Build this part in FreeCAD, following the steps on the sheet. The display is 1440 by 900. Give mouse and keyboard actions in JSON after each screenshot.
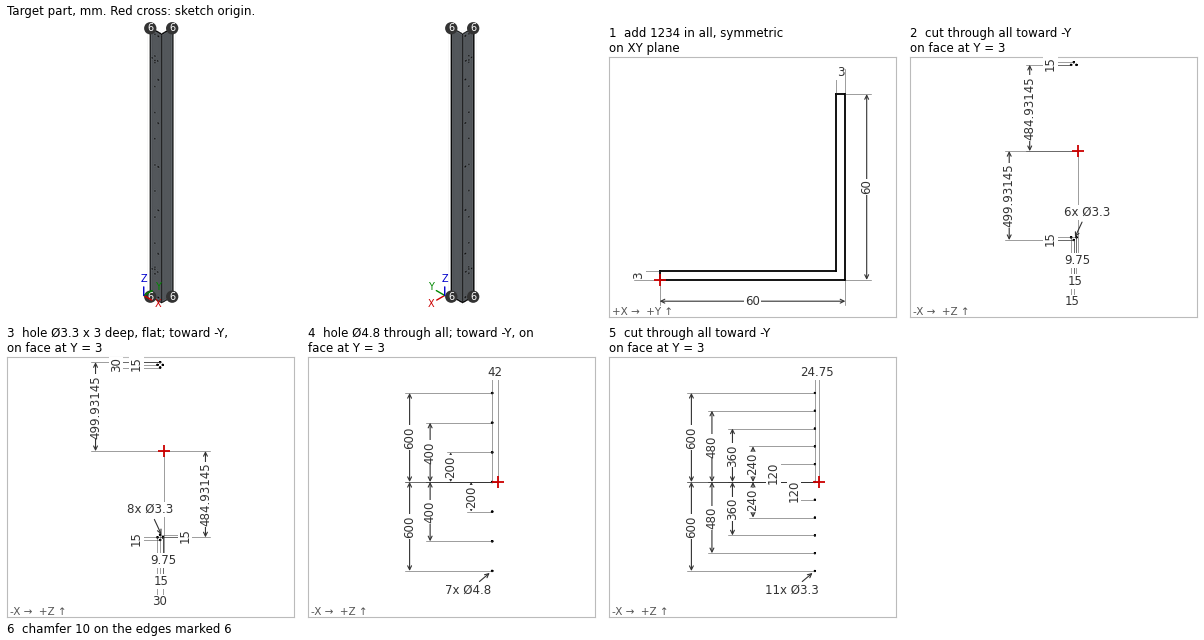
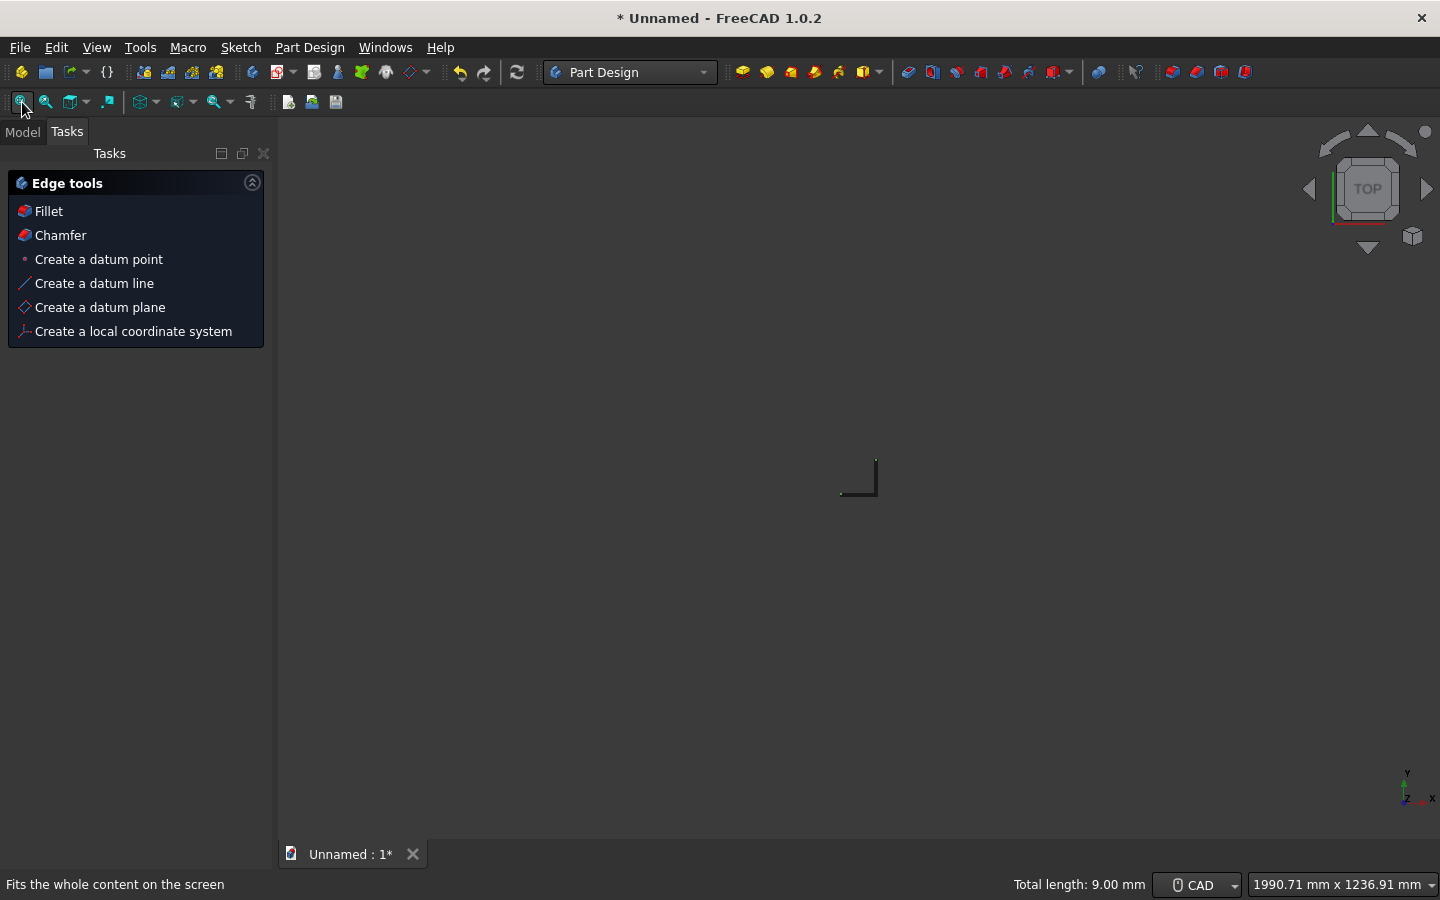
{"action": "left_click", "coordinate": [22, 102]}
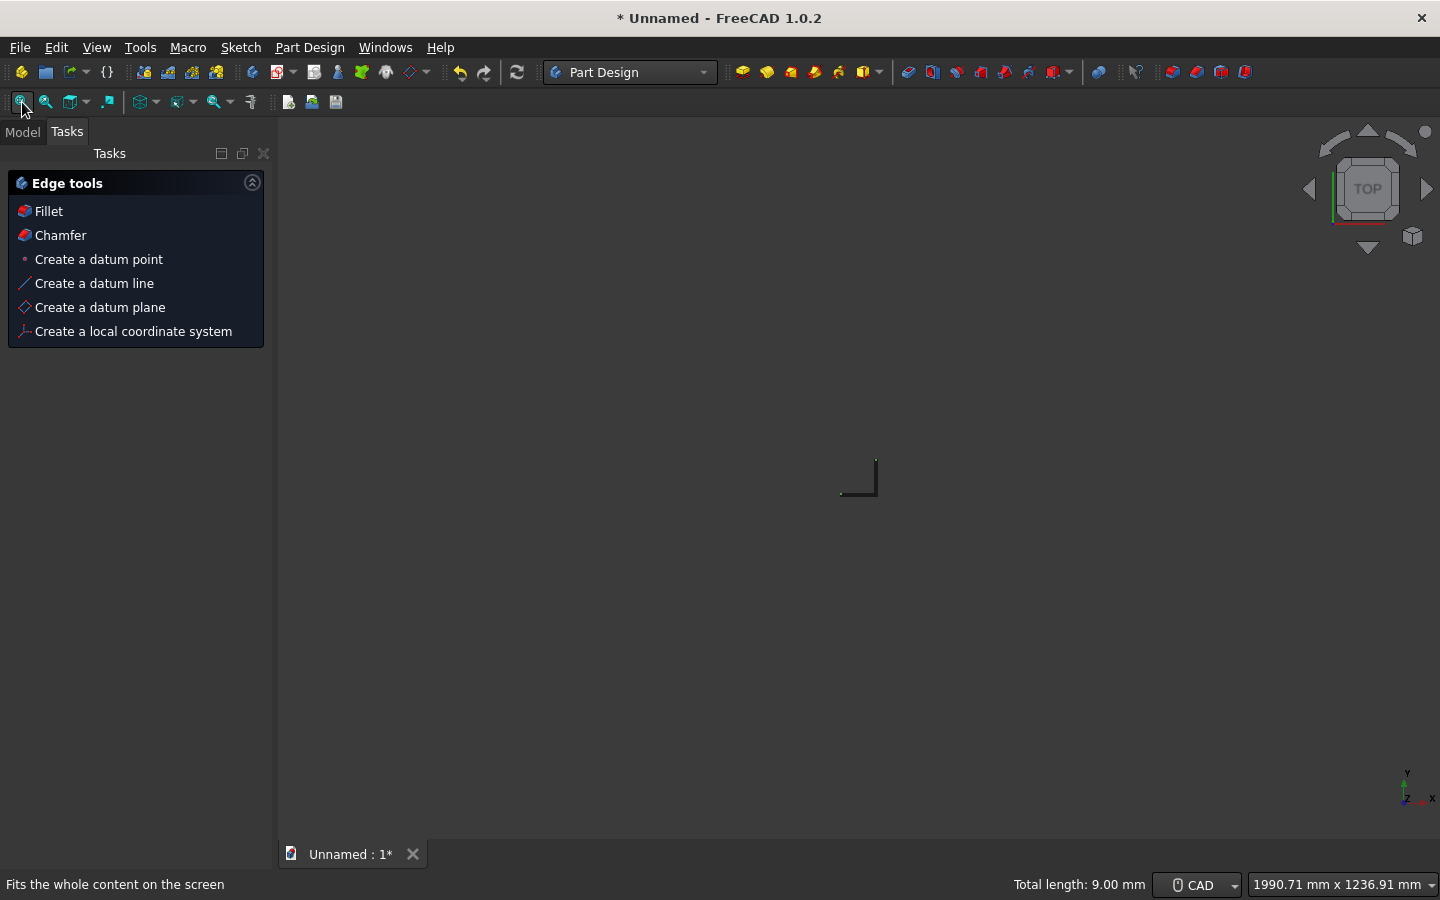
{"action": "scroll", "coordinate": [876, 459], "scroll_direction": "up", "scroll_amount": 15}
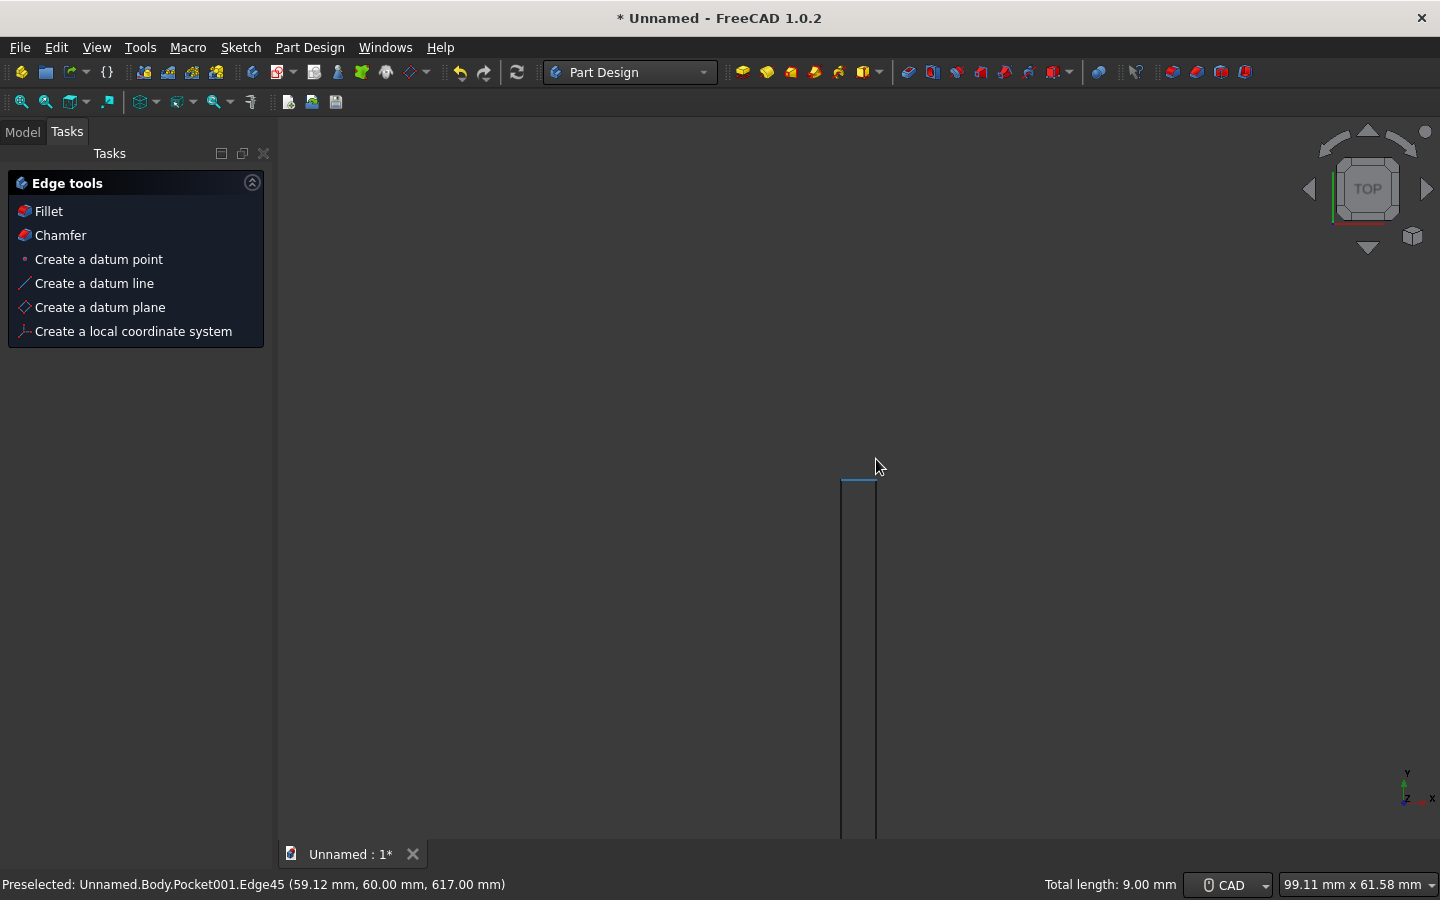
{"action": "left_click", "coordinate": [22, 102]}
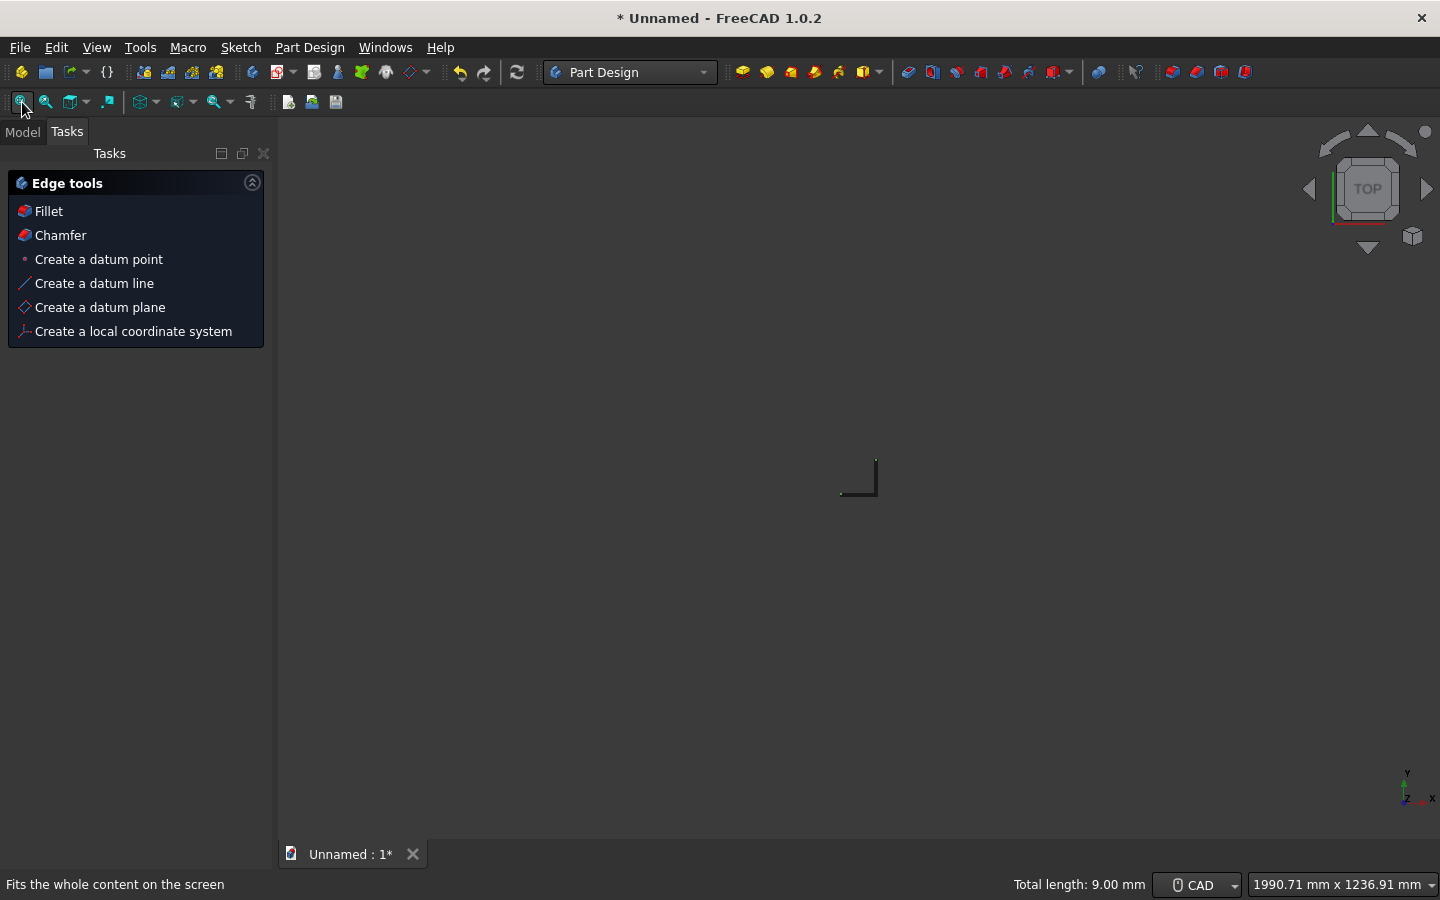
{"action": "key", "text": "1"}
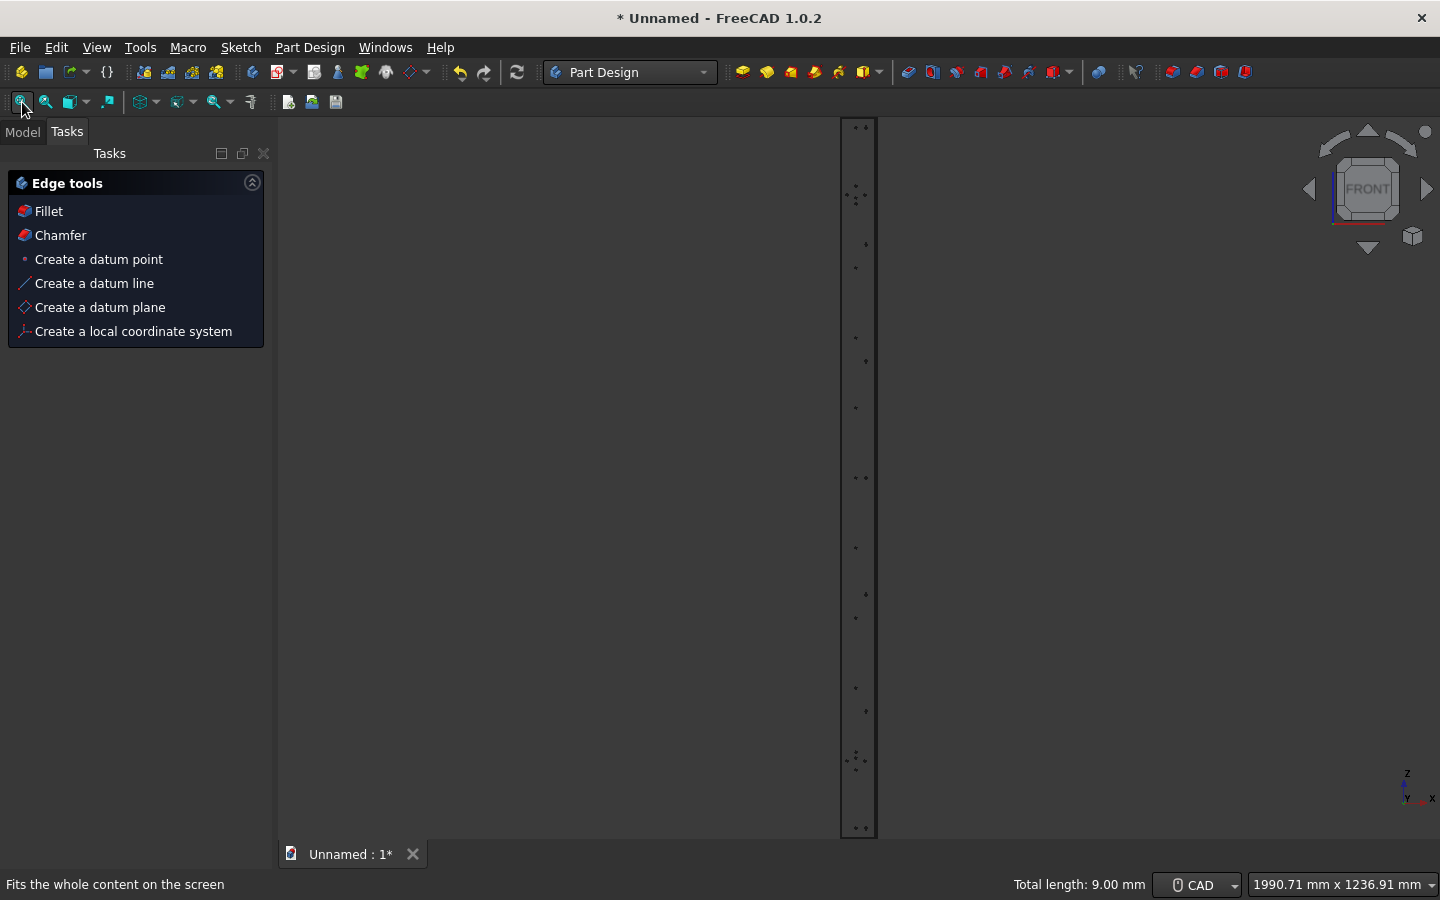
{"action": "key", "text": "3"}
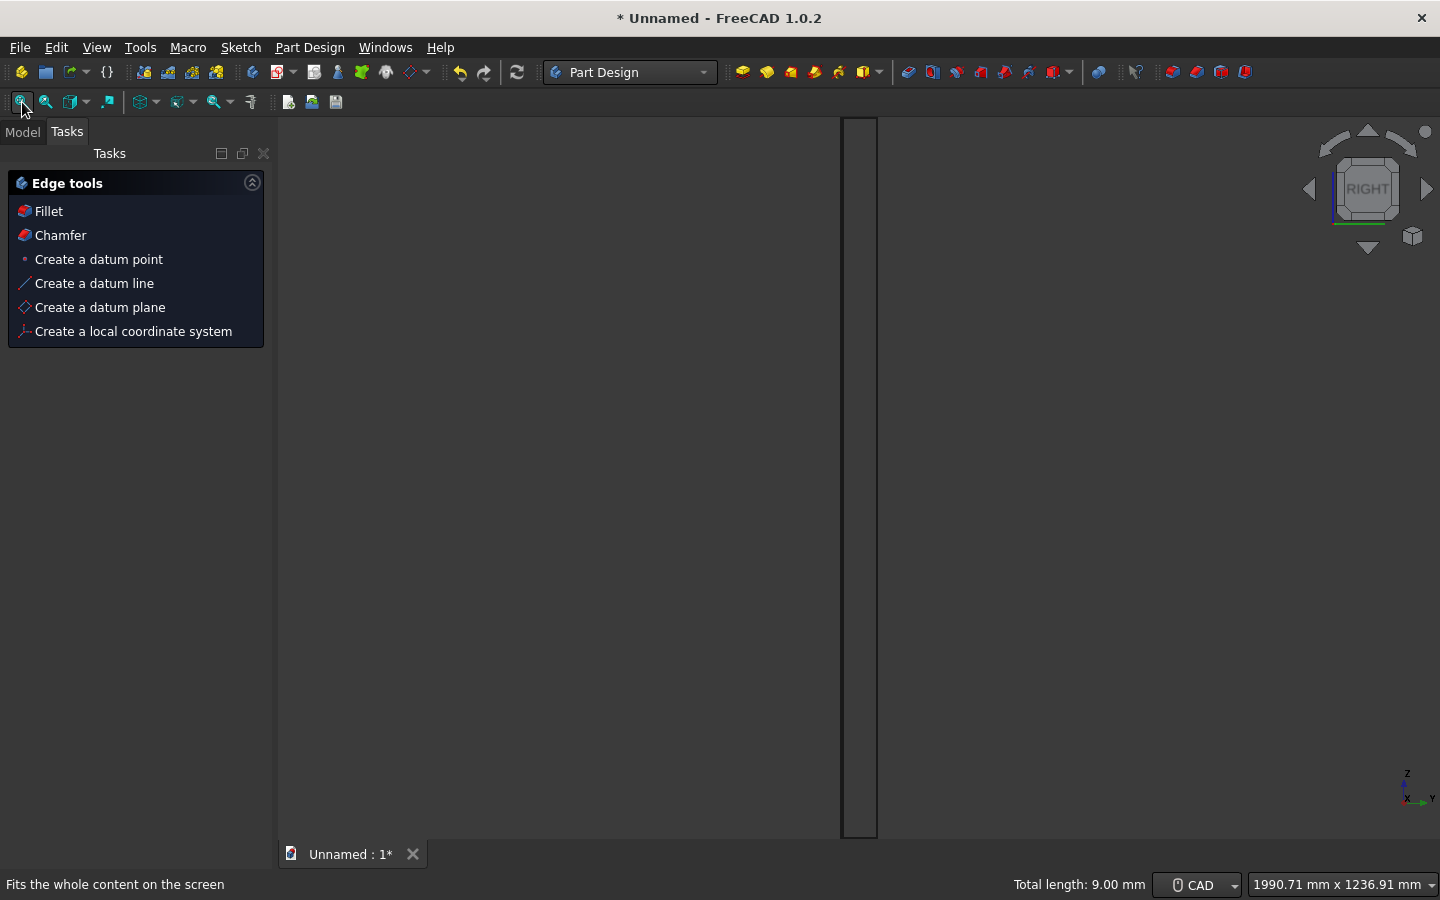
{"action": "key", "text": "5"}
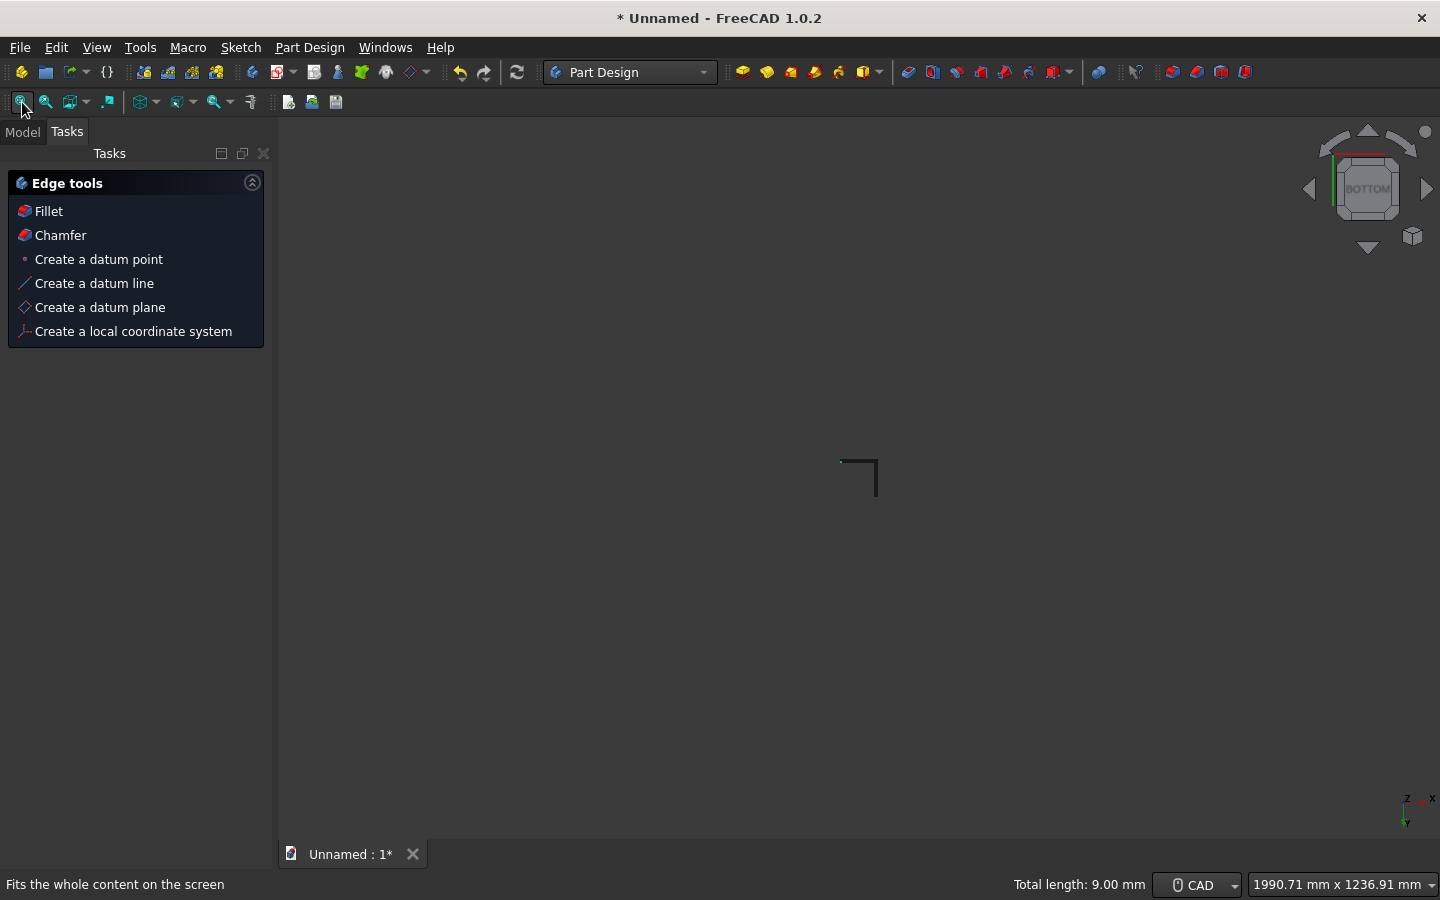
{"action": "left_click", "coordinate": [22, 102]}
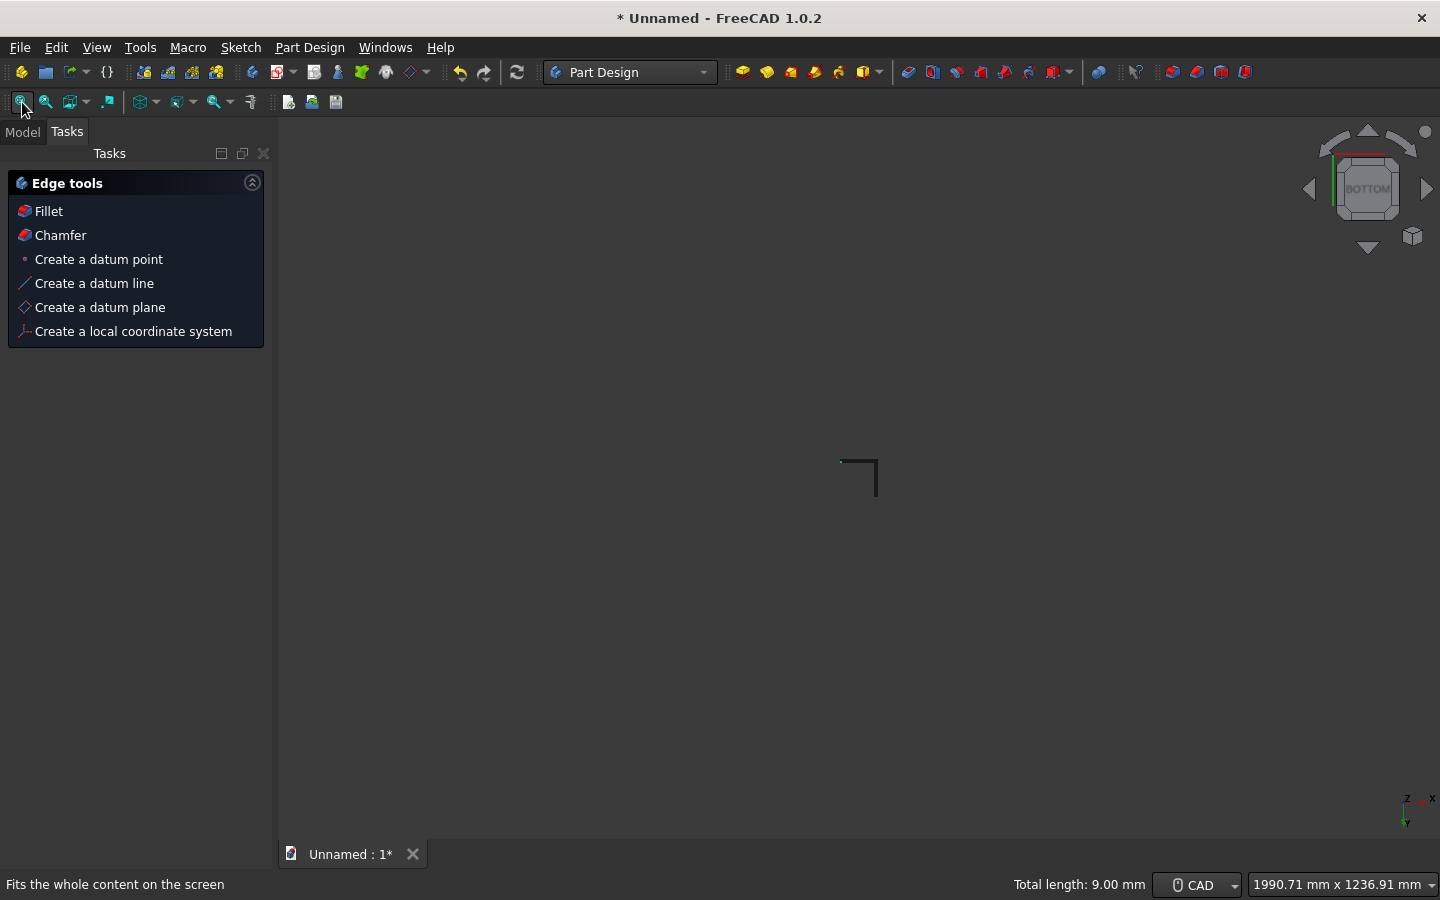
{"action": "scroll", "coordinate": [876, 495], "scroll_direction": "up", "scroll_amount": 15}